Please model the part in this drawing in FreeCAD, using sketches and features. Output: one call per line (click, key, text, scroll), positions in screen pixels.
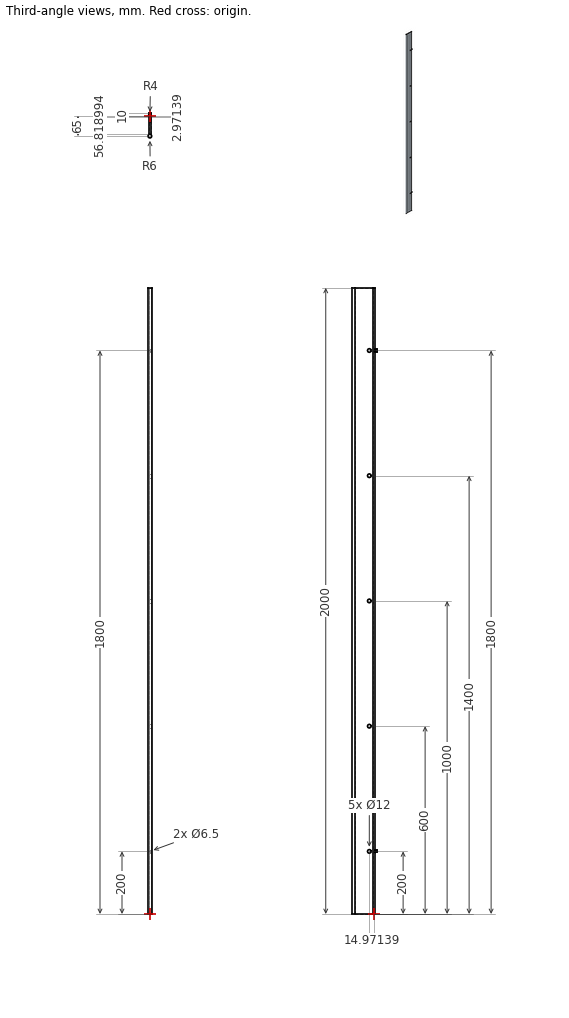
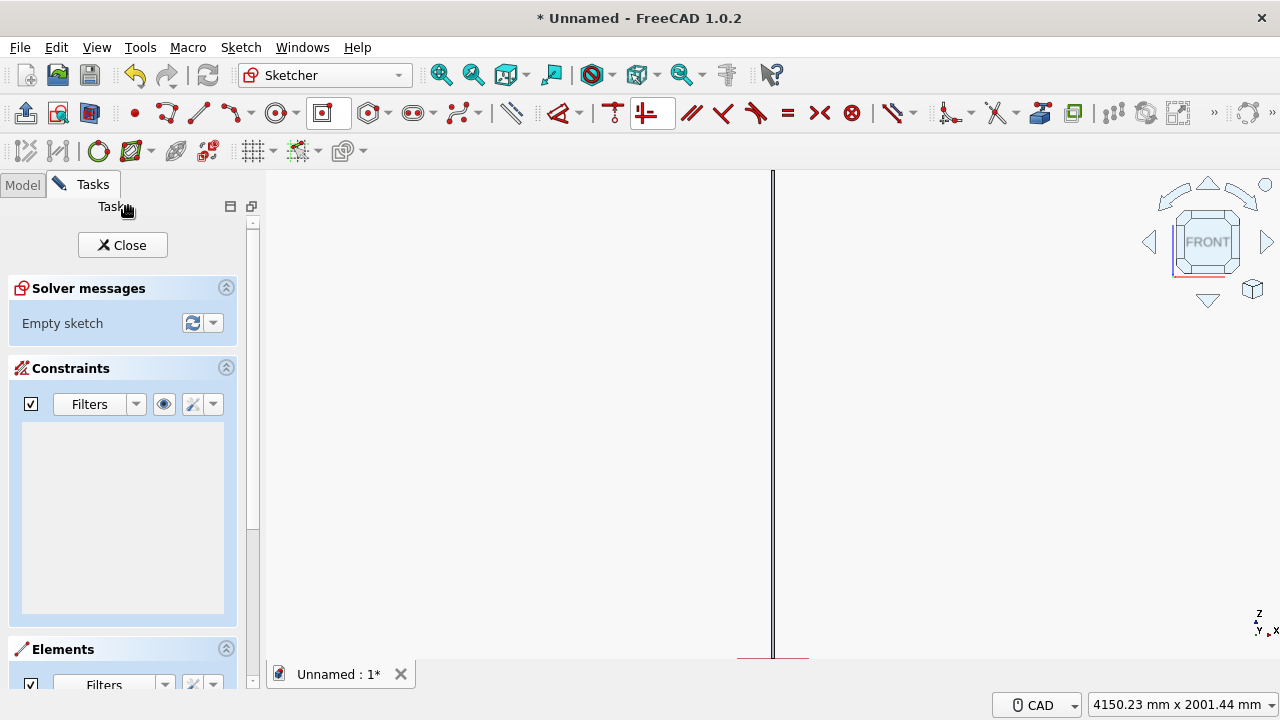
key(q)
key(s)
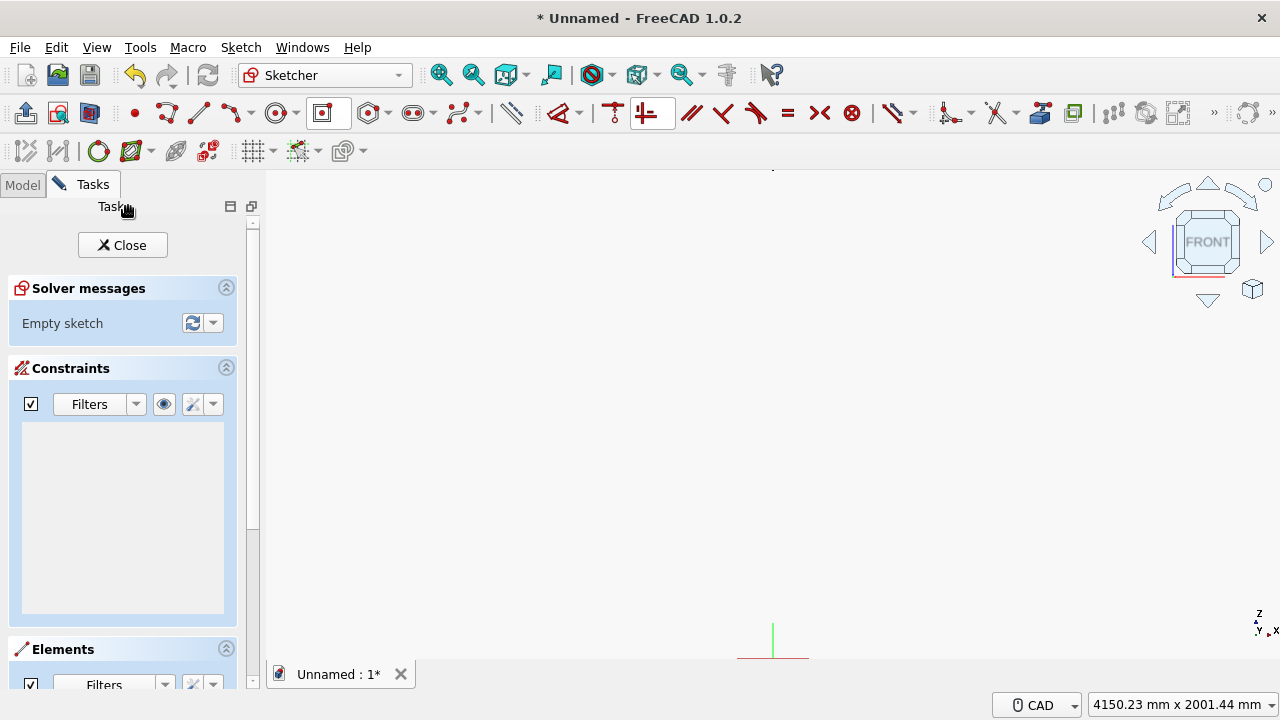
scroll(565, 366, down, 2)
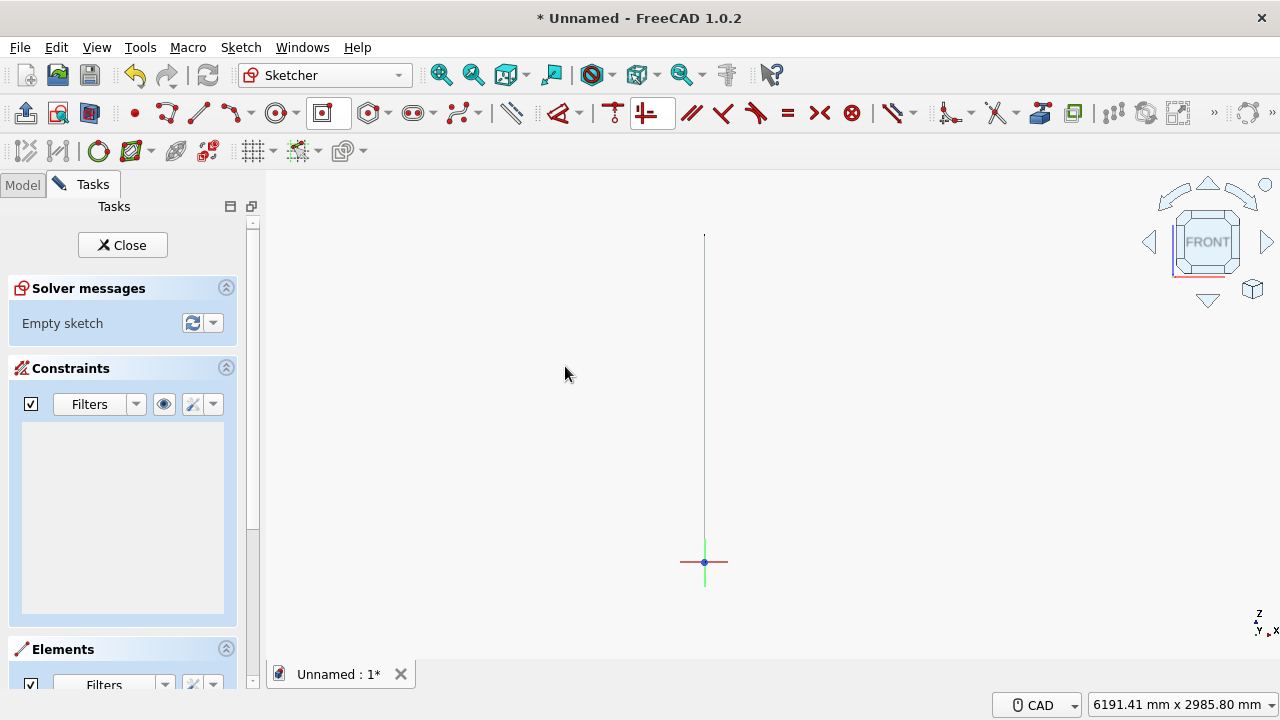
click(276, 114)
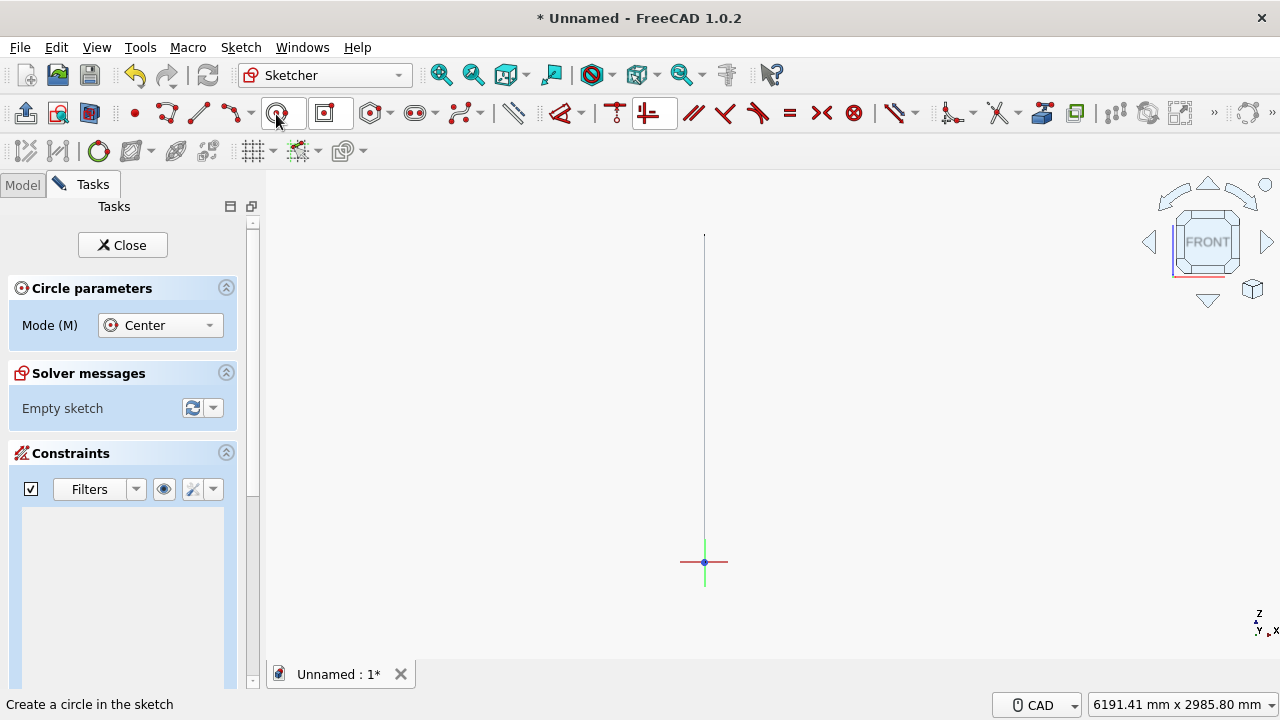
scroll(705, 530, up, 19)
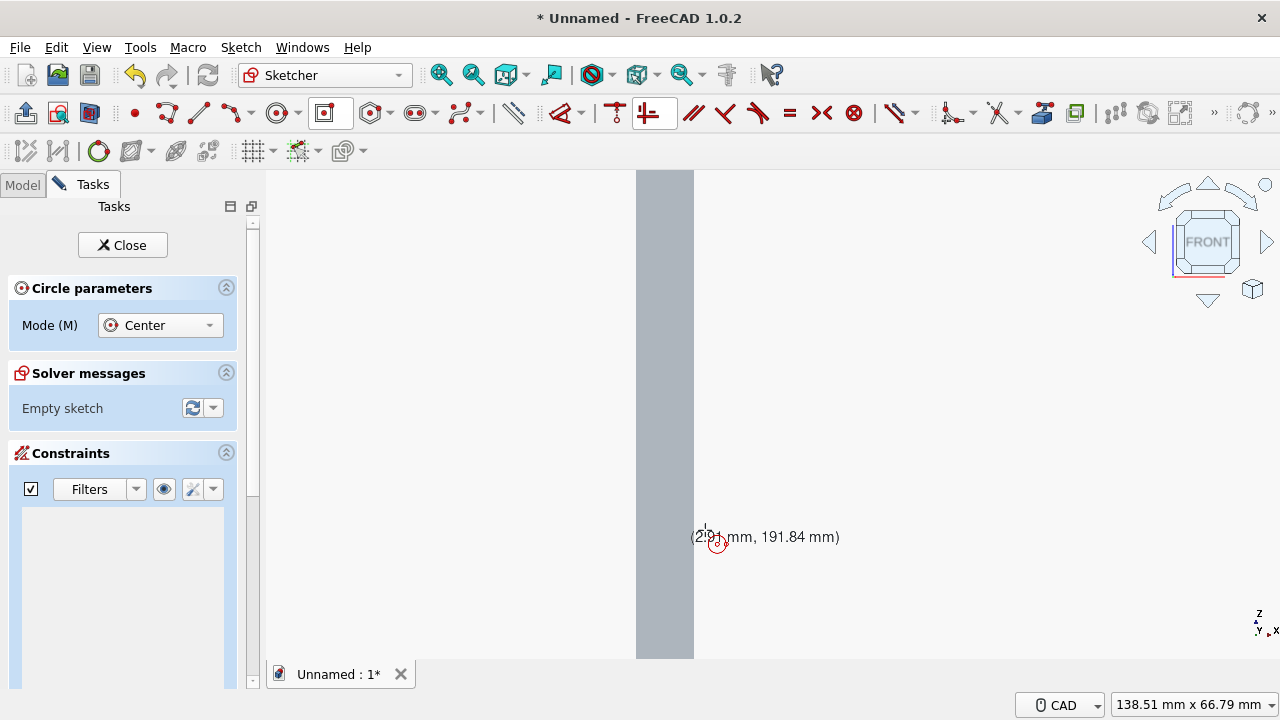
scroll(706, 557, down, 18)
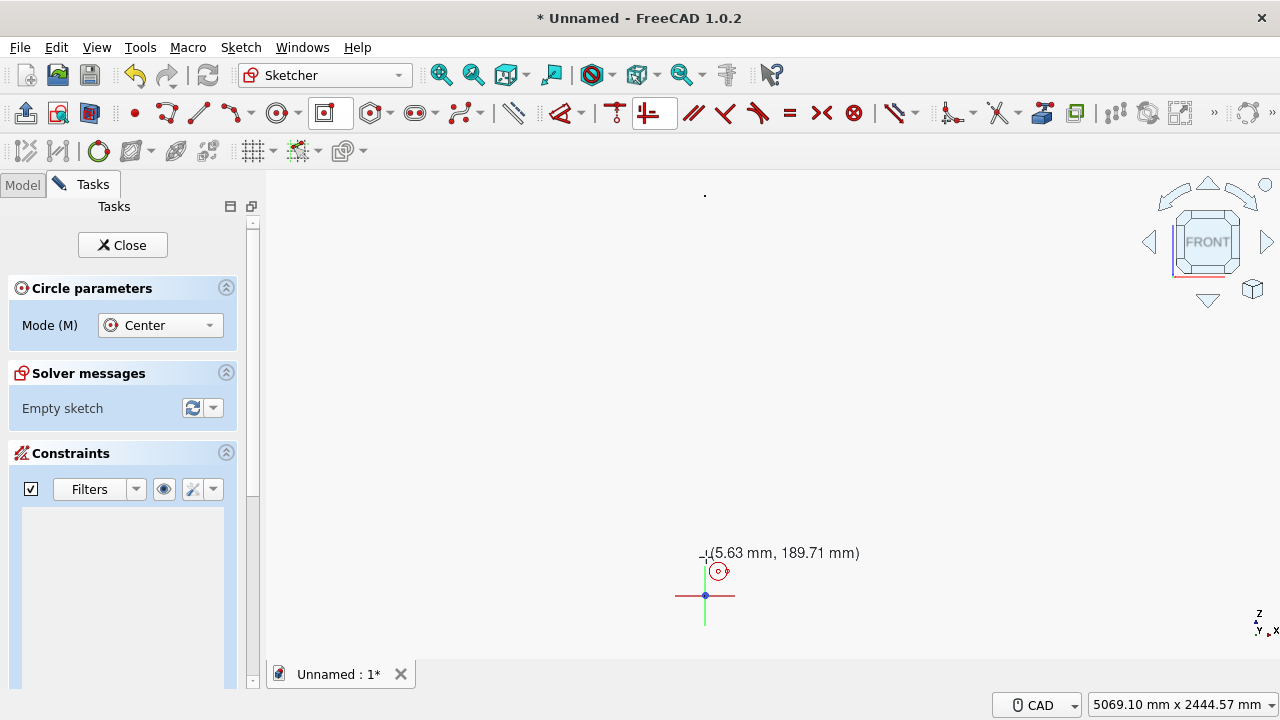
click(705, 556)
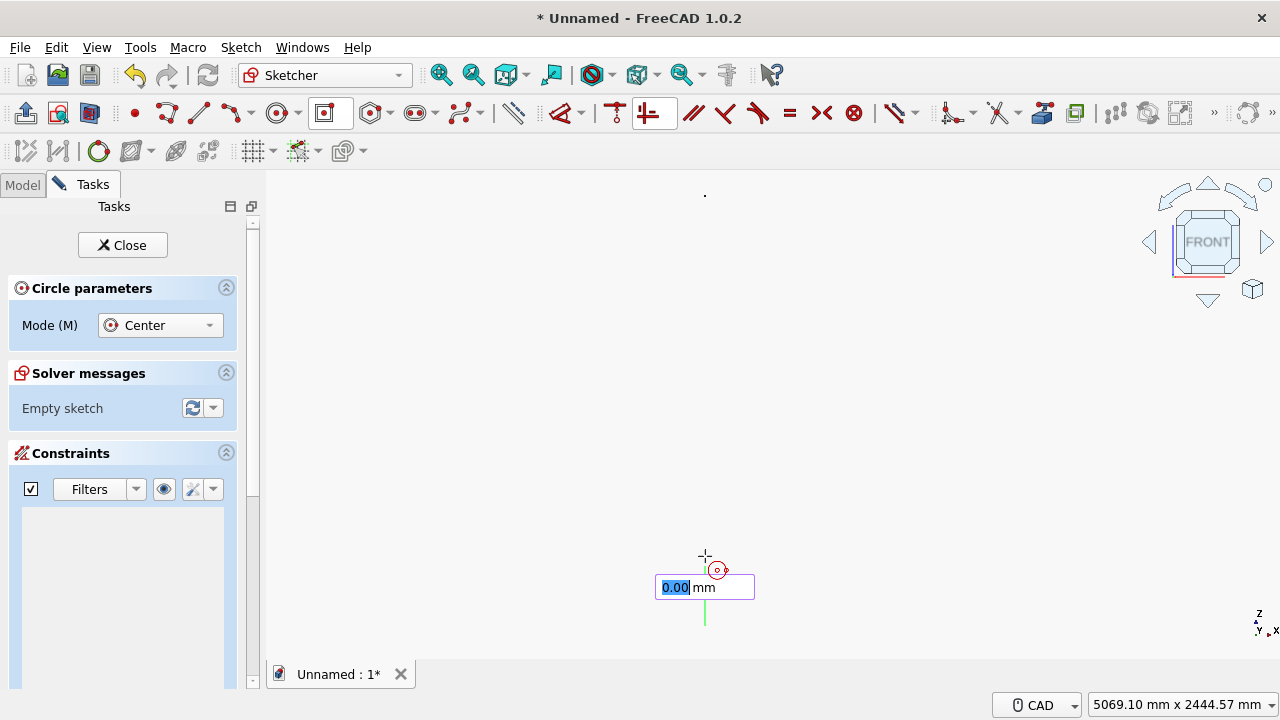
scroll(706, 556, up, 17)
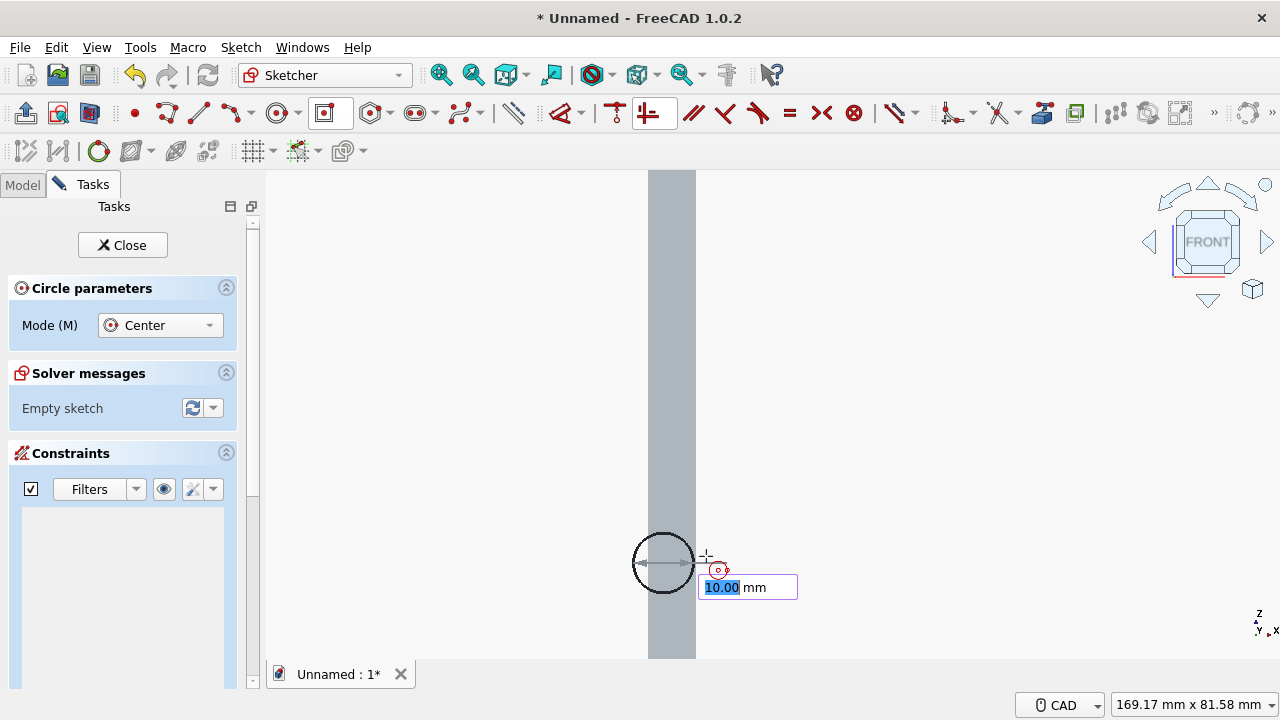
click(691, 519)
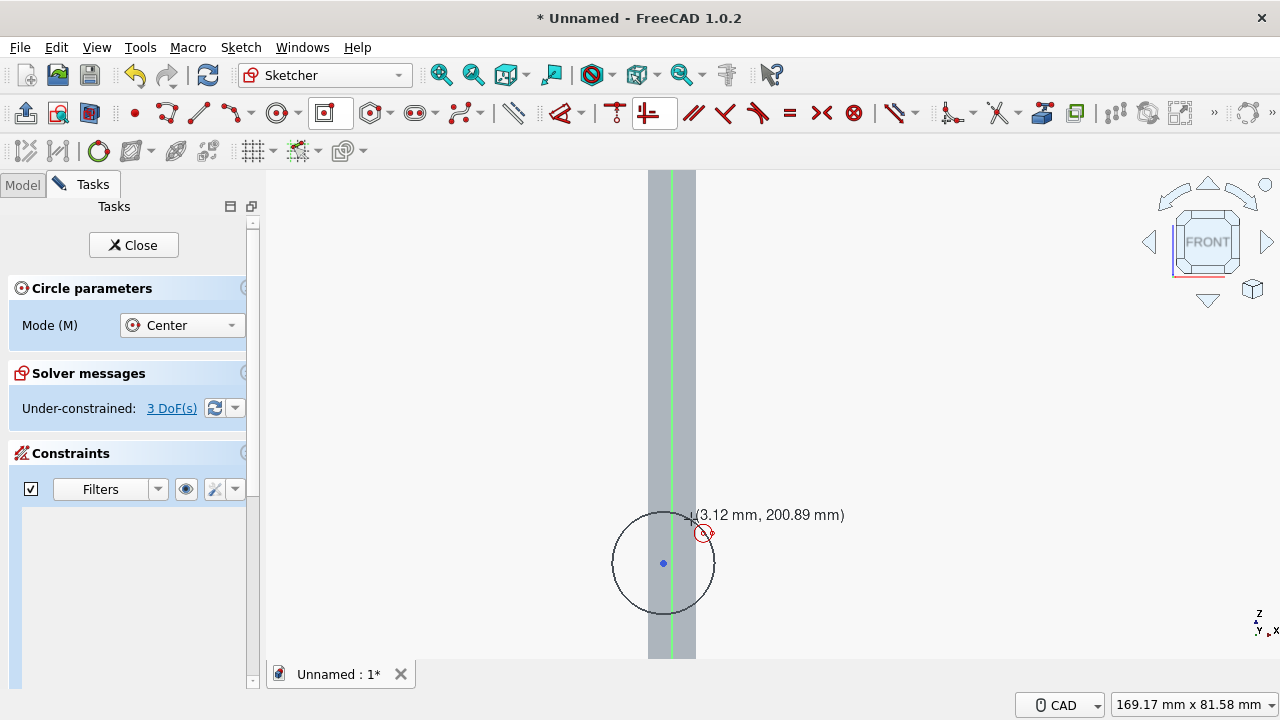
scroll(706, 556, down, 17)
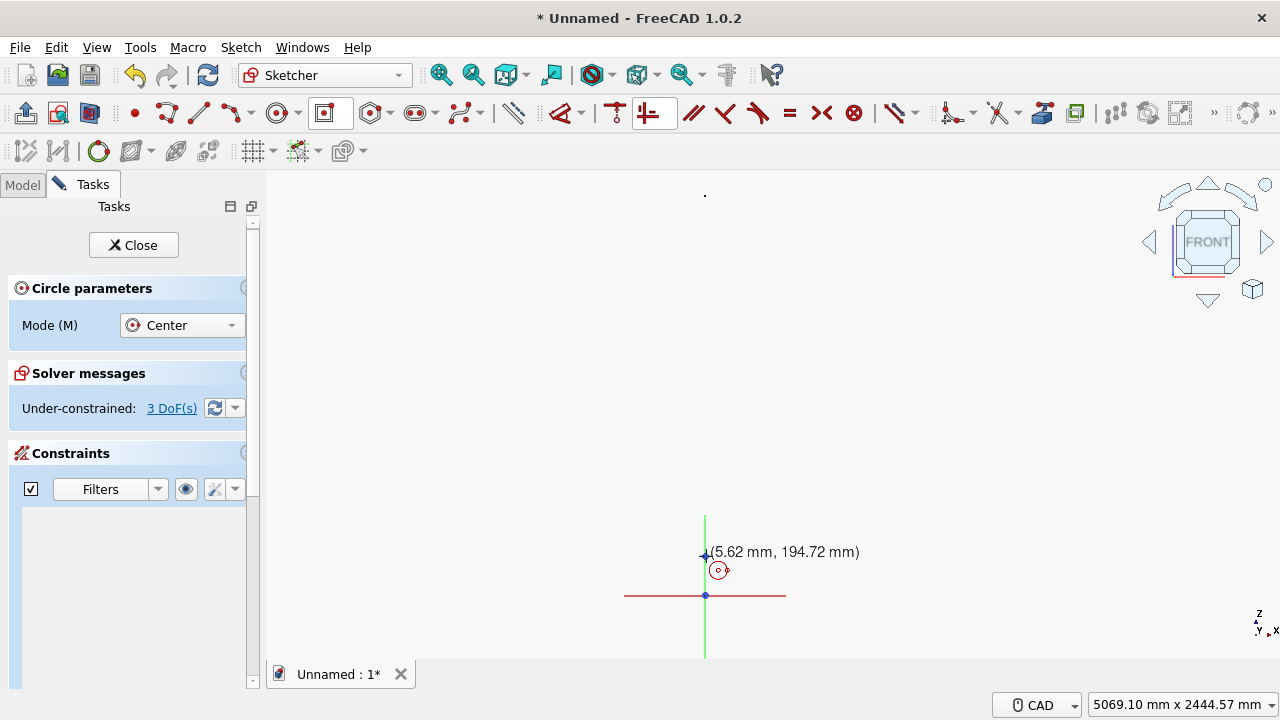
scroll(705, 236, up, 18)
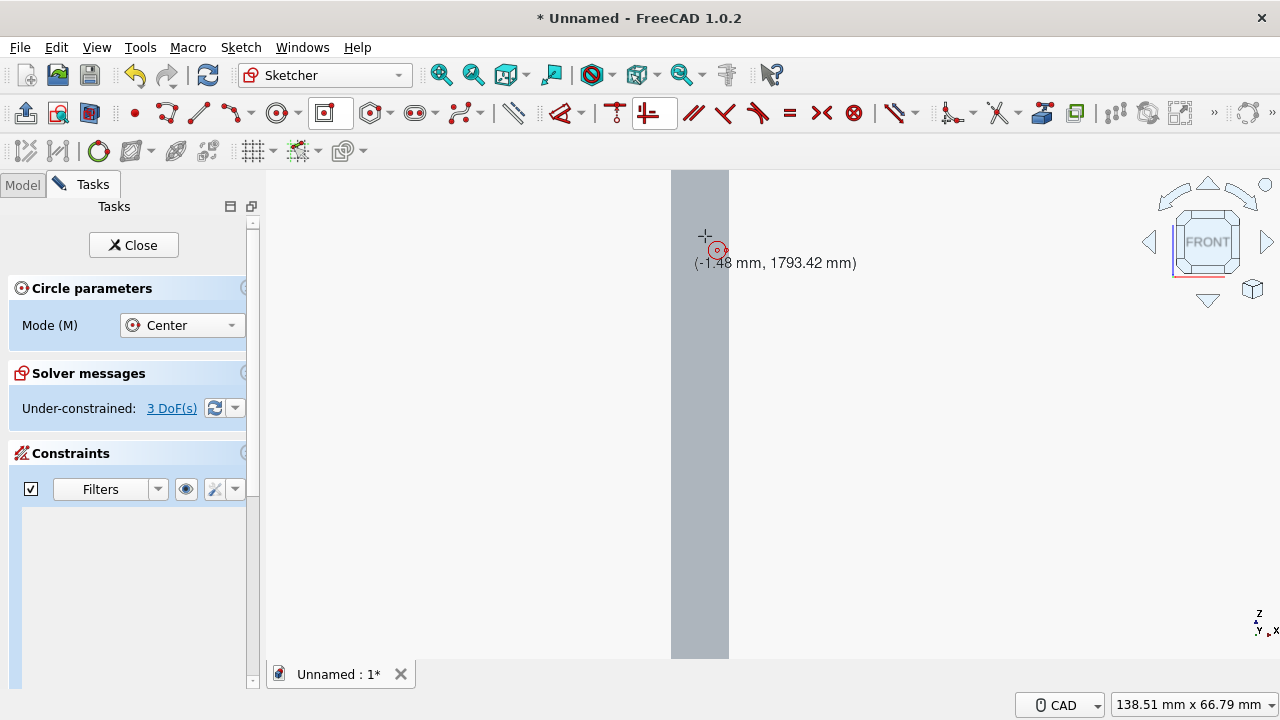
scroll(705, 235, down, 18)